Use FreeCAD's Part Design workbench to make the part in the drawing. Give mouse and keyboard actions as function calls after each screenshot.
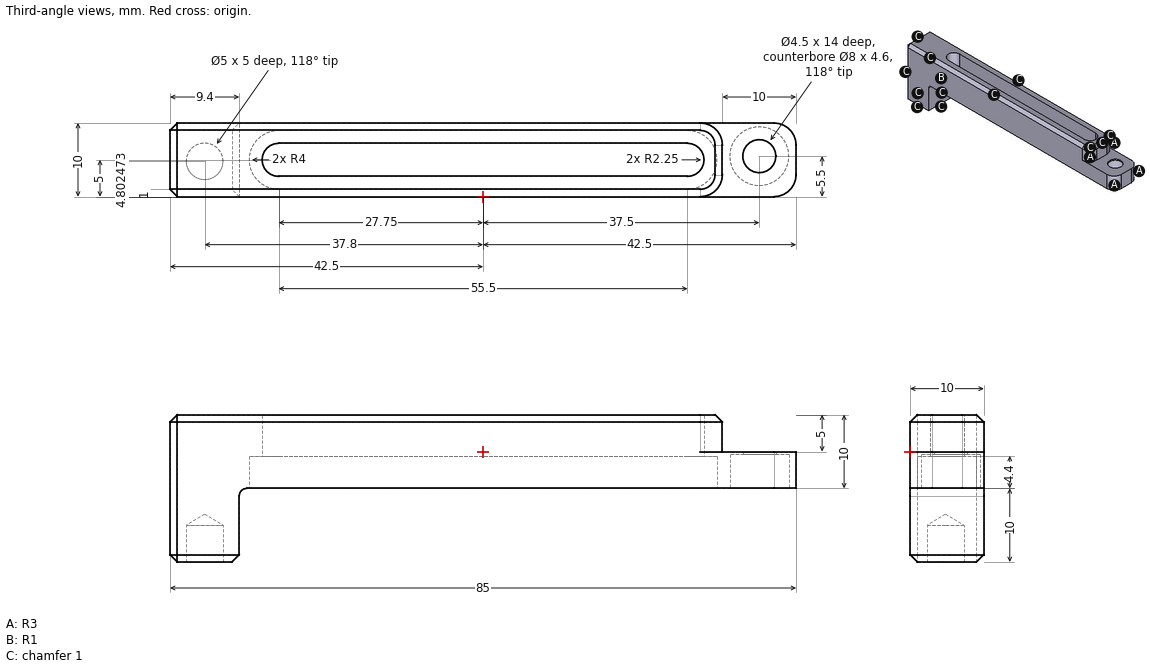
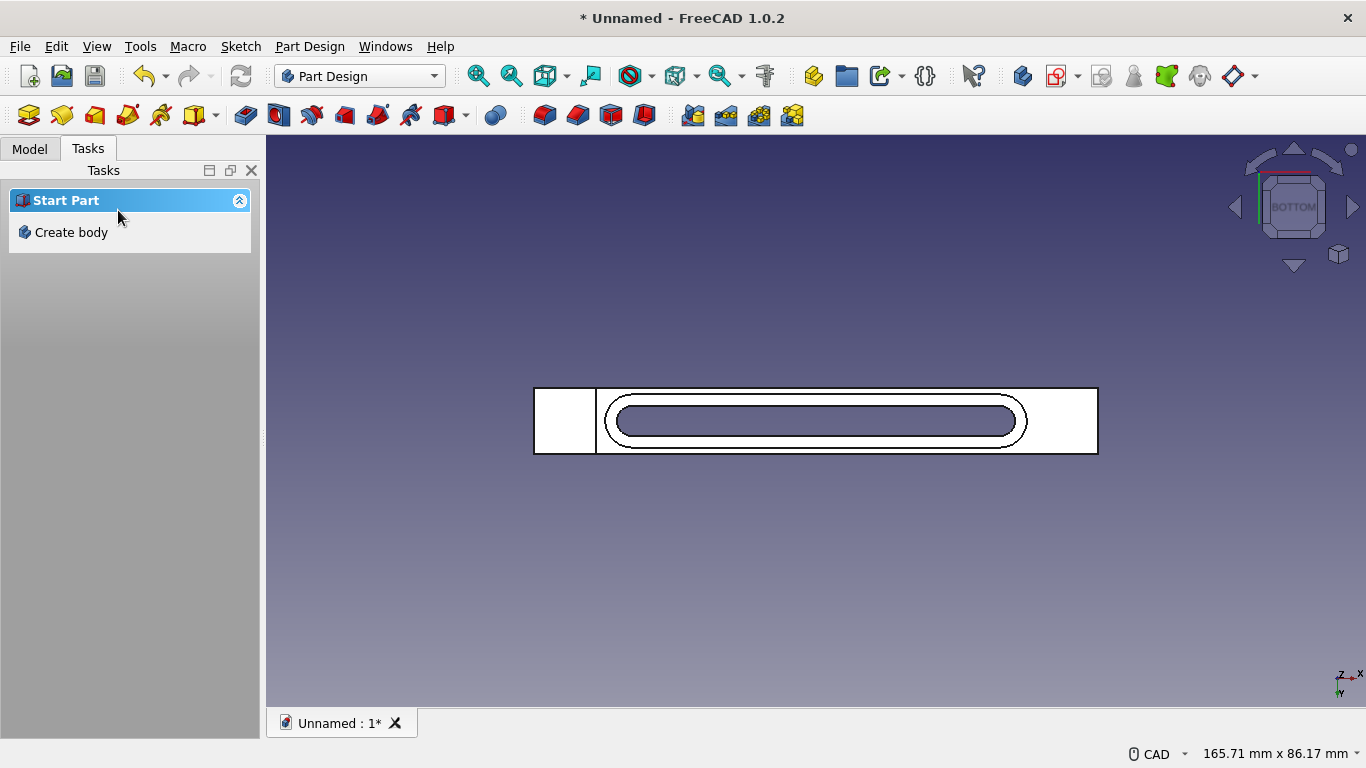
key(0)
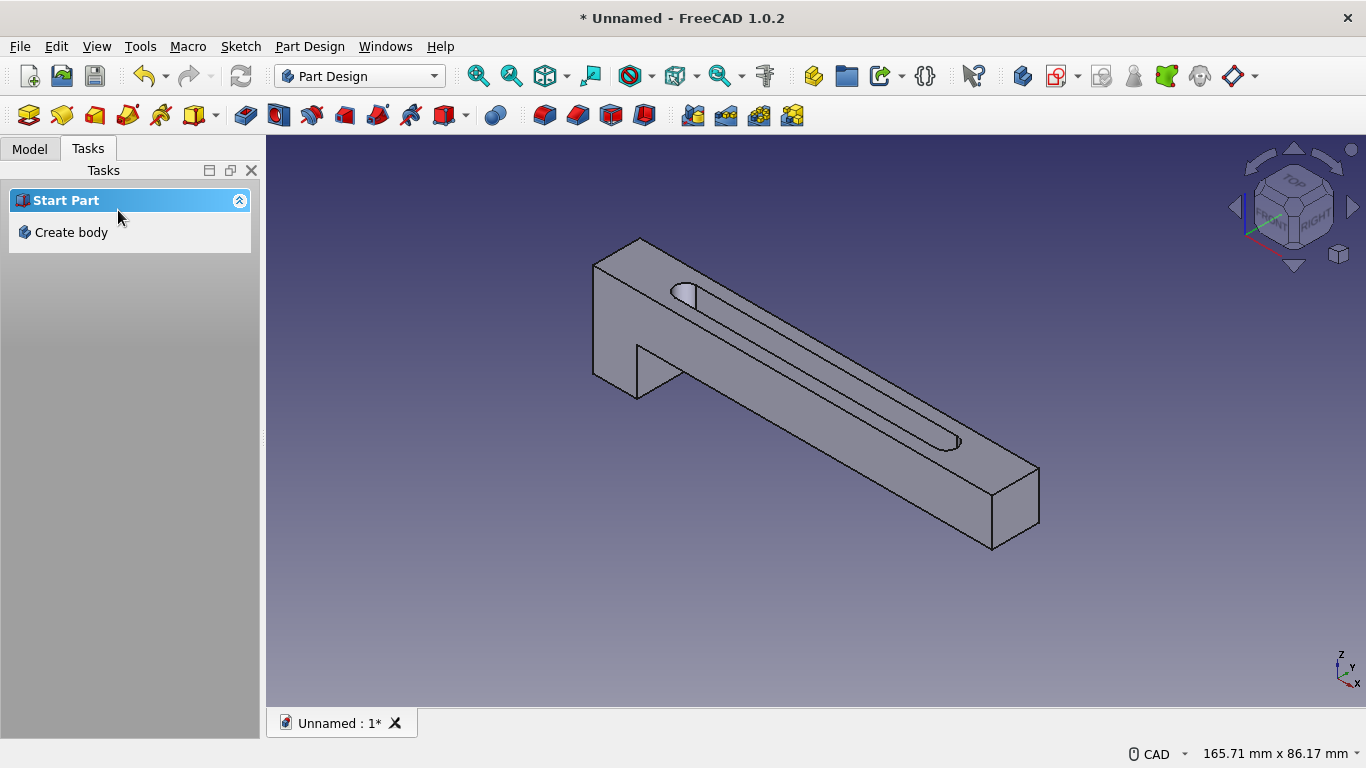
click(987, 465)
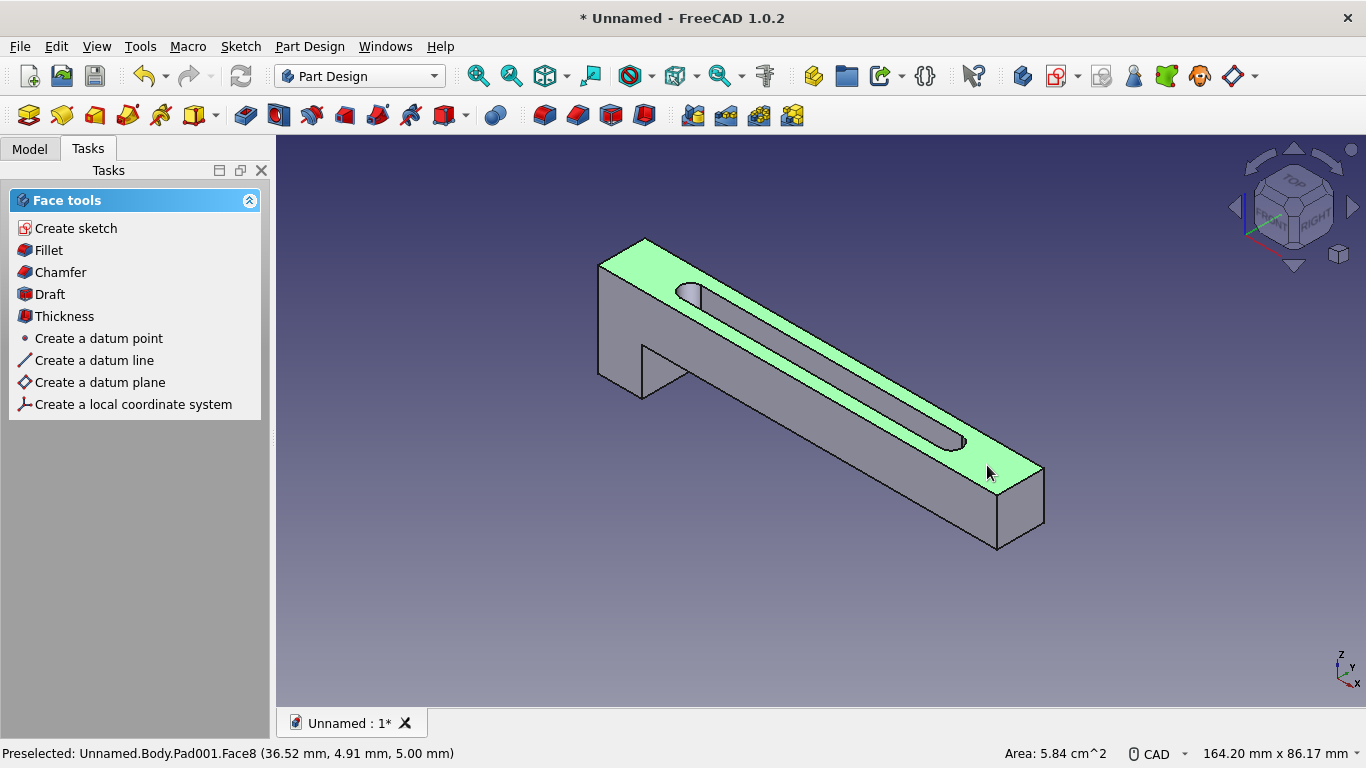
click(1056, 76)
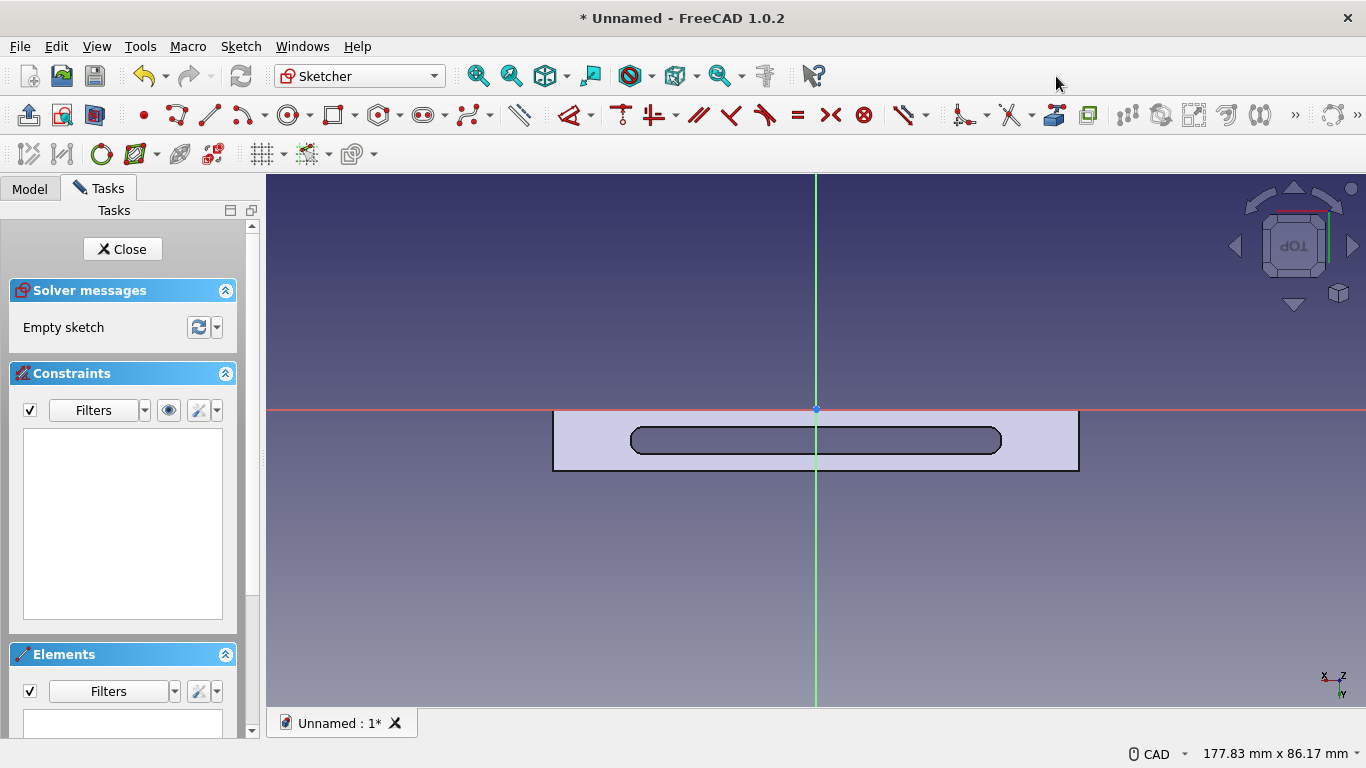
scroll(543, 441, up, 8)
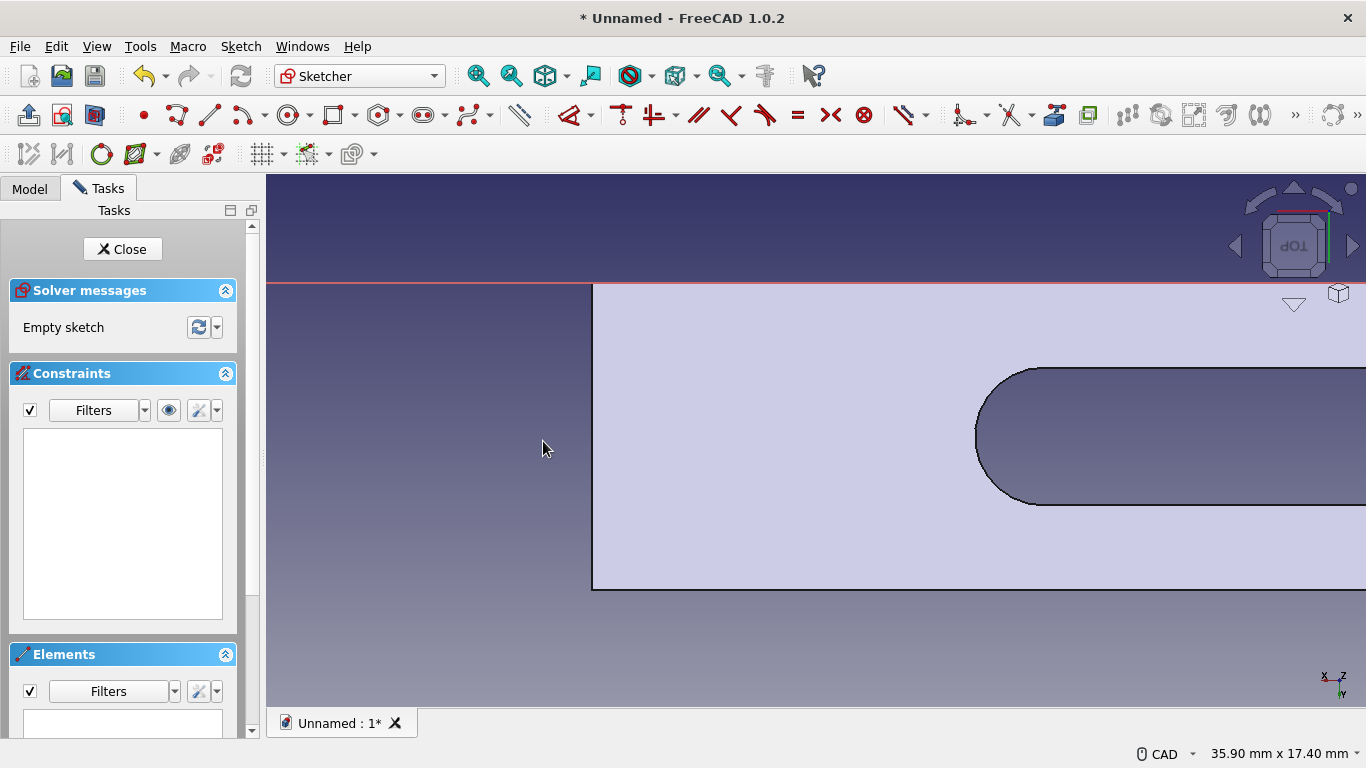
key(g)
key(r)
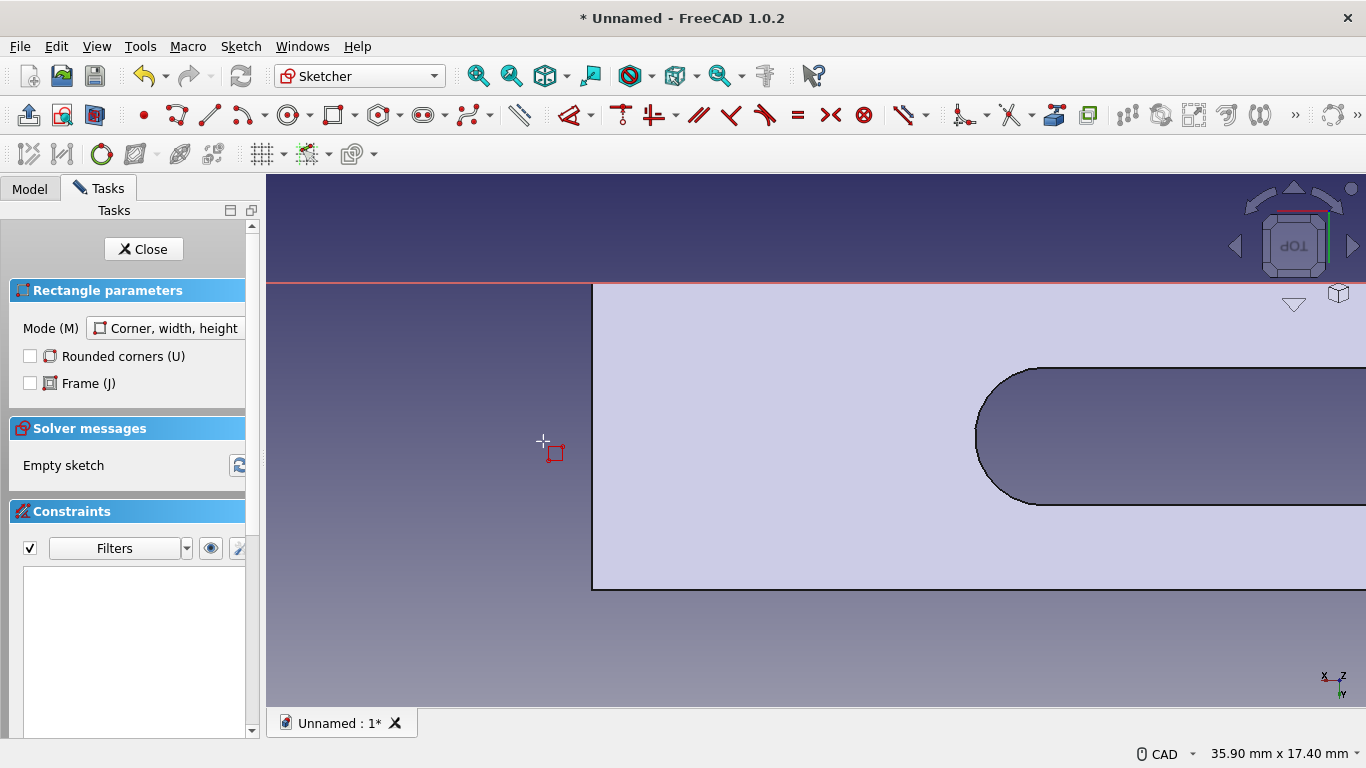
click(592, 283)
click(898, 590)
key(Escape)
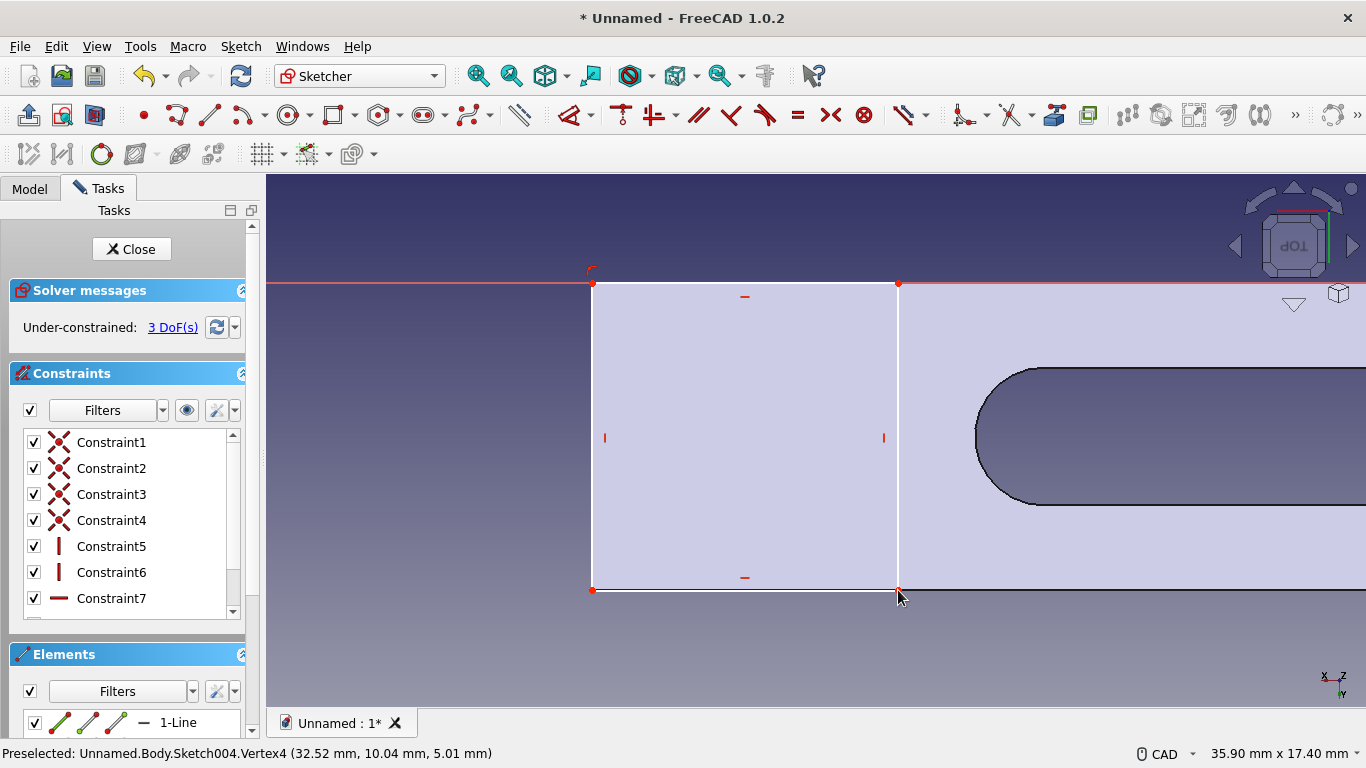
key(d)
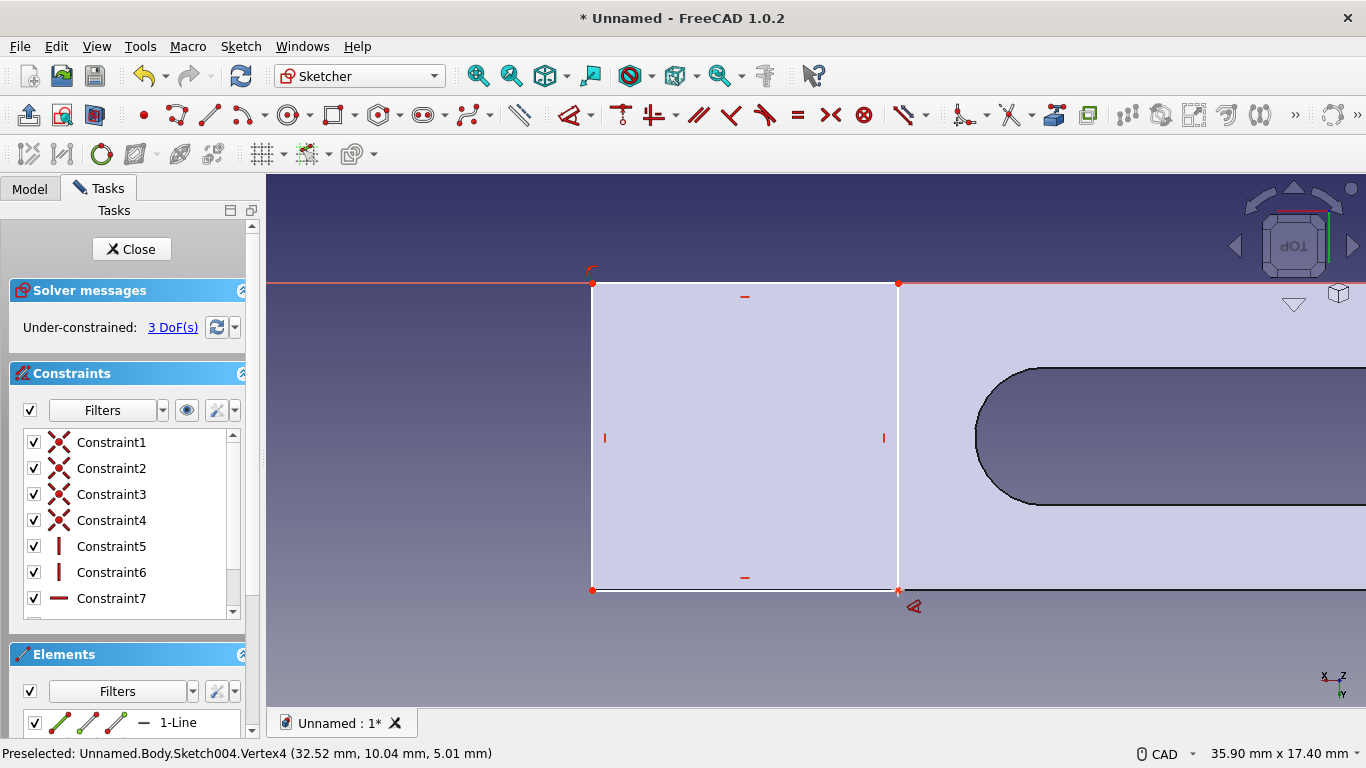
click(592, 376)
click(558, 437)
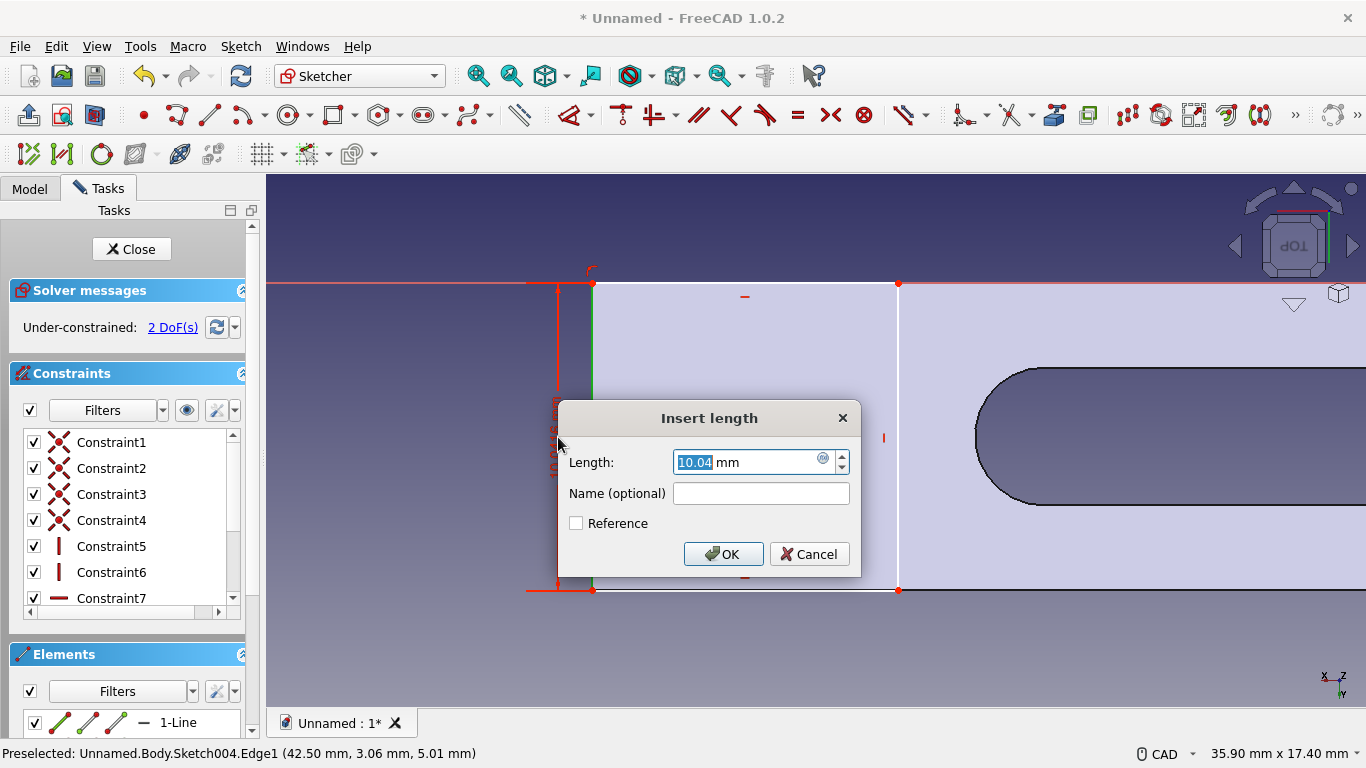
text(10)
key(Return)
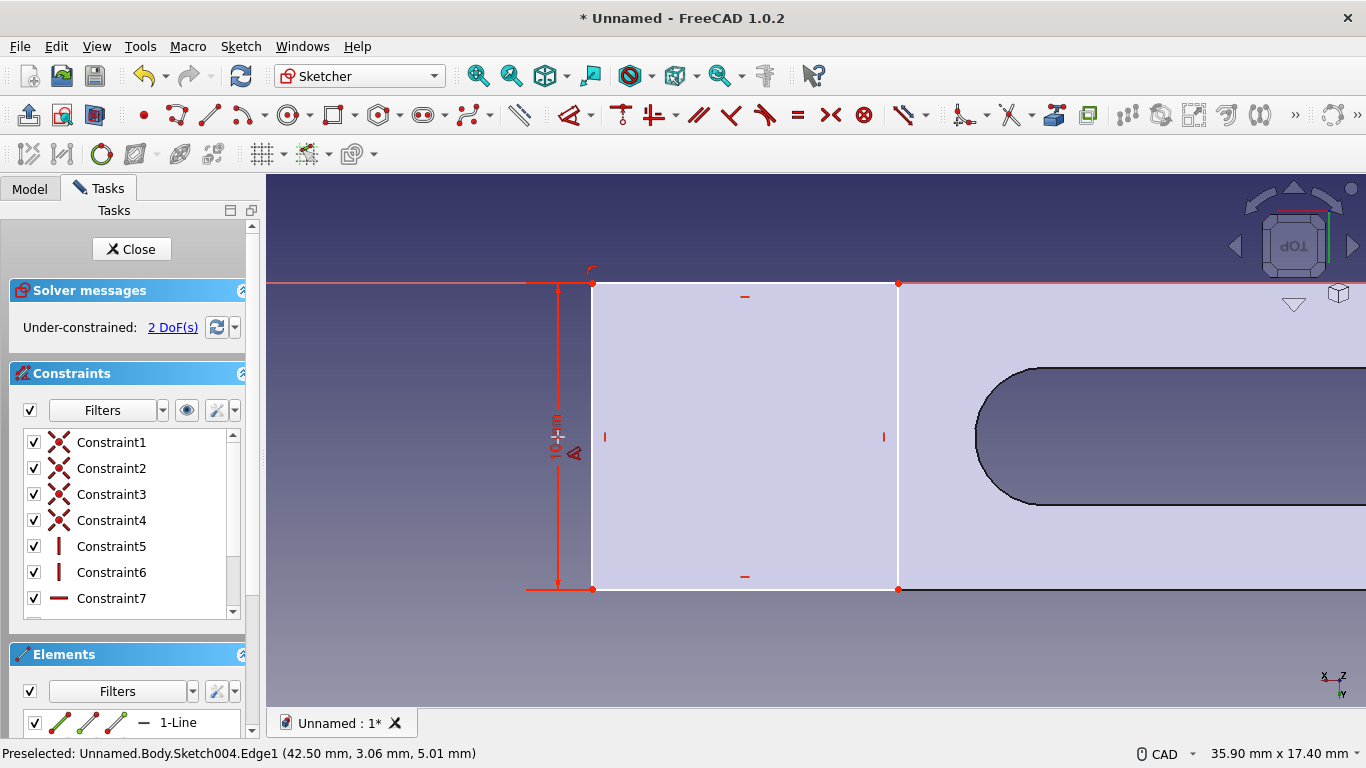
click(684, 590)
click(745, 624)